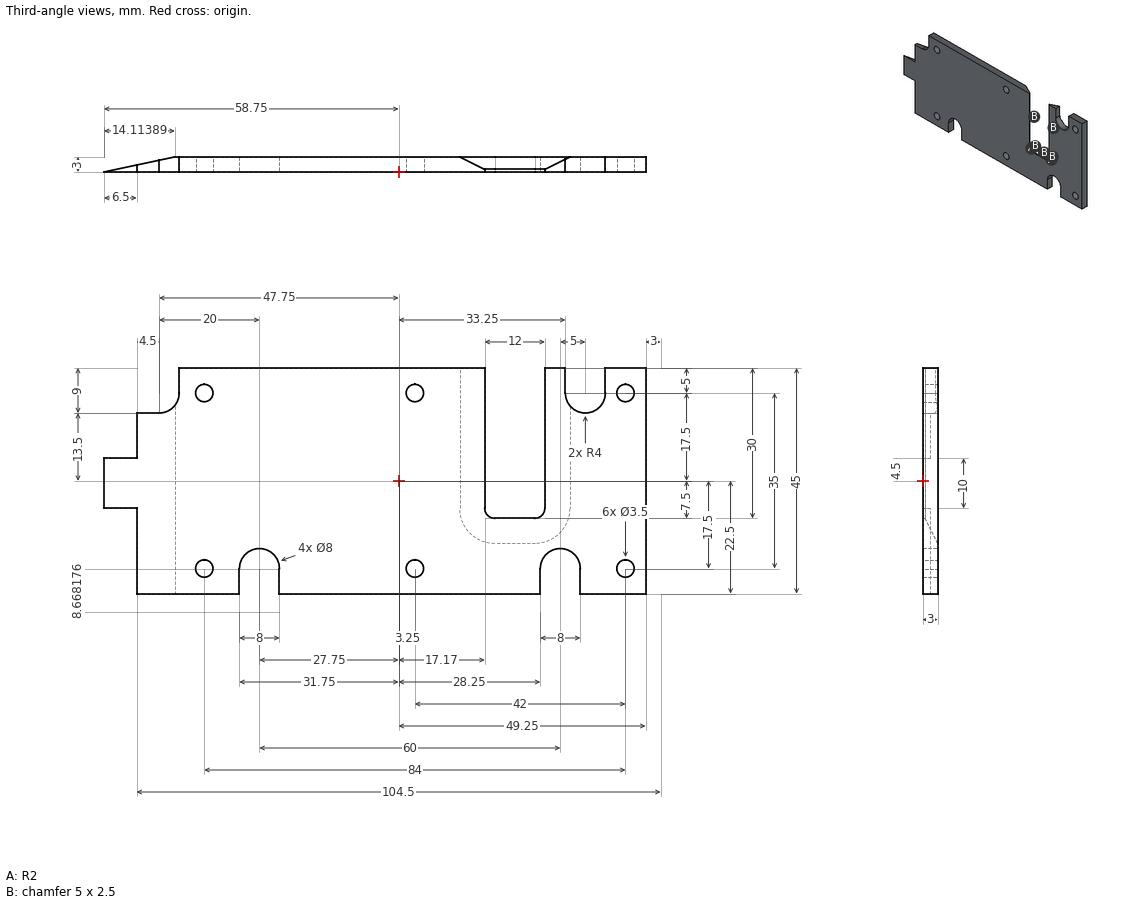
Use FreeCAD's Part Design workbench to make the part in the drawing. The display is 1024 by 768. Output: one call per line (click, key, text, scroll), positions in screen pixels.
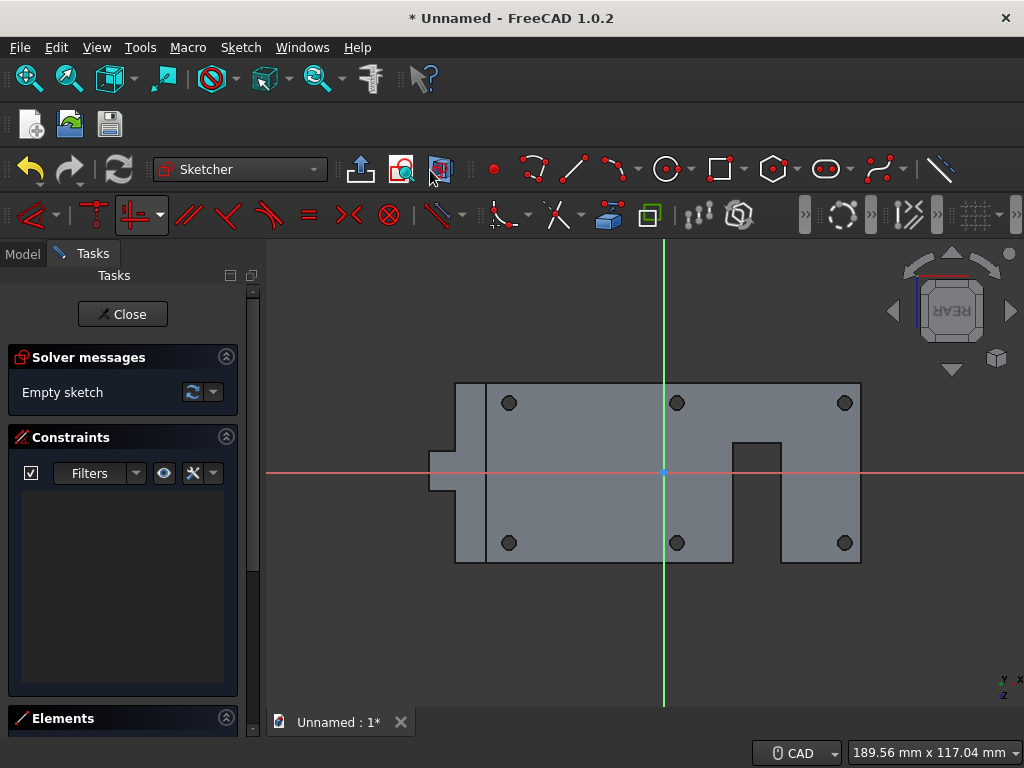
key(g)
key(c)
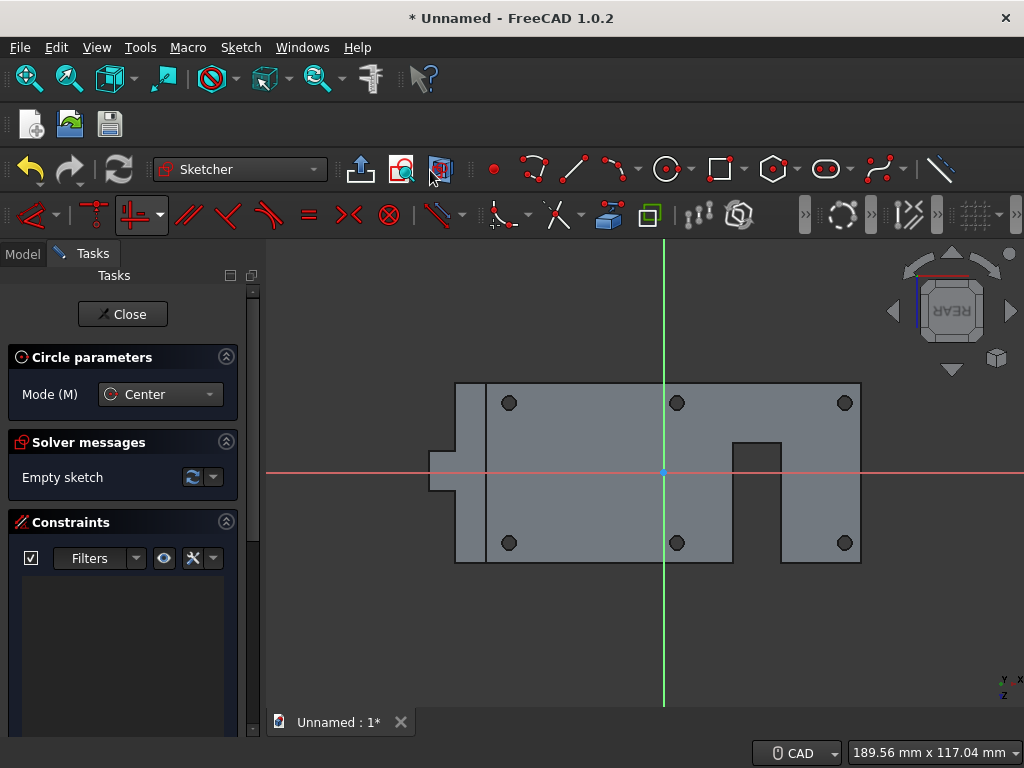
scroll(553, 403, up, 2)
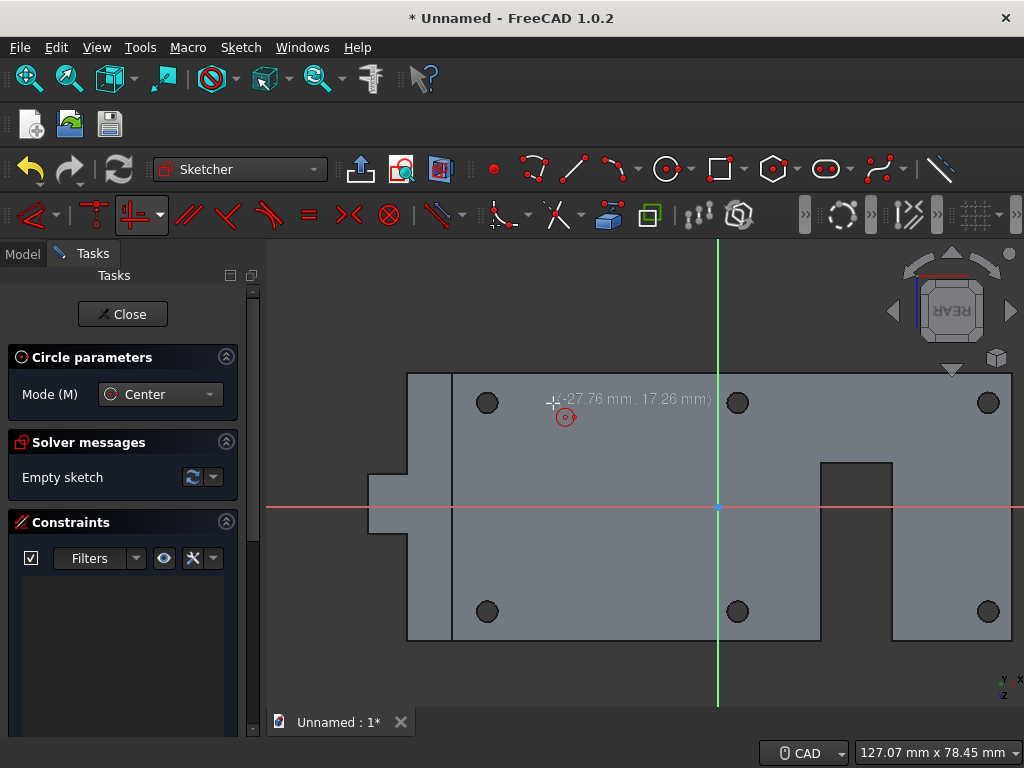
click(553, 403)
move(570, 386)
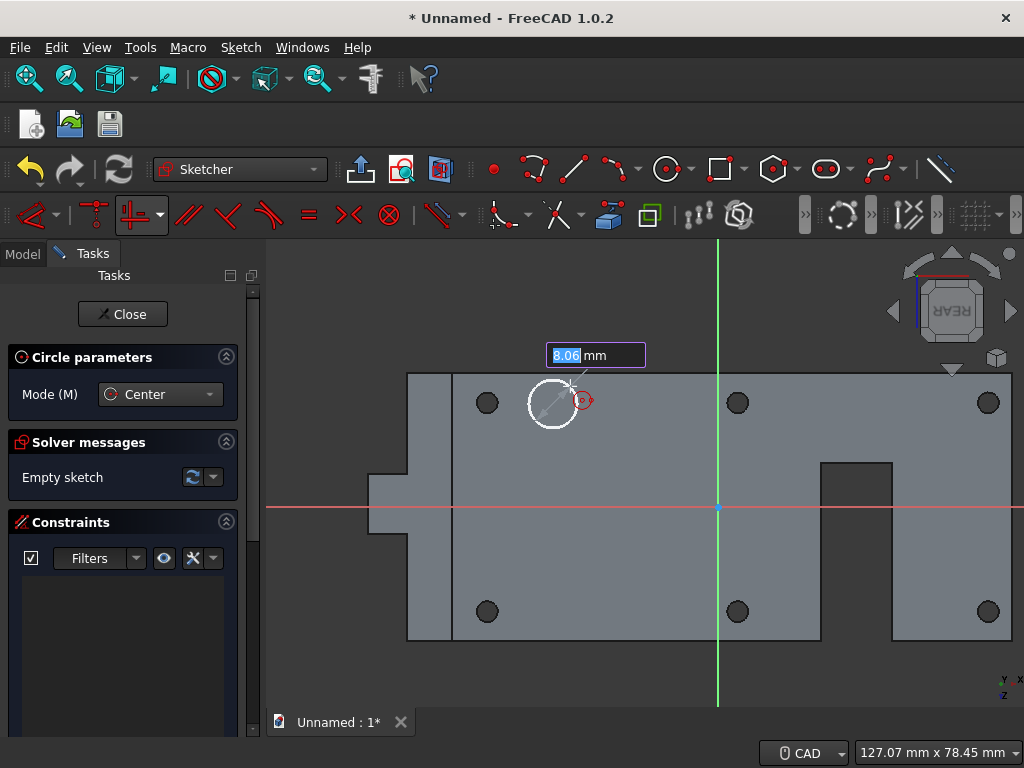
text(8)
key(Return)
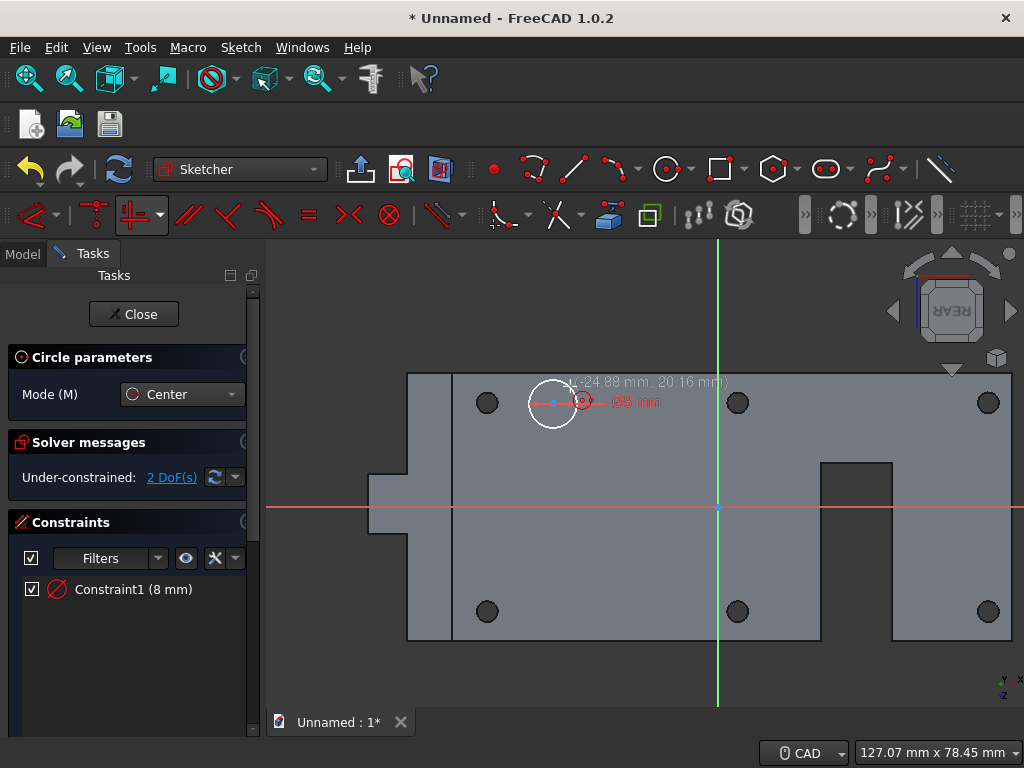
click(434, 612)
move(450, 595)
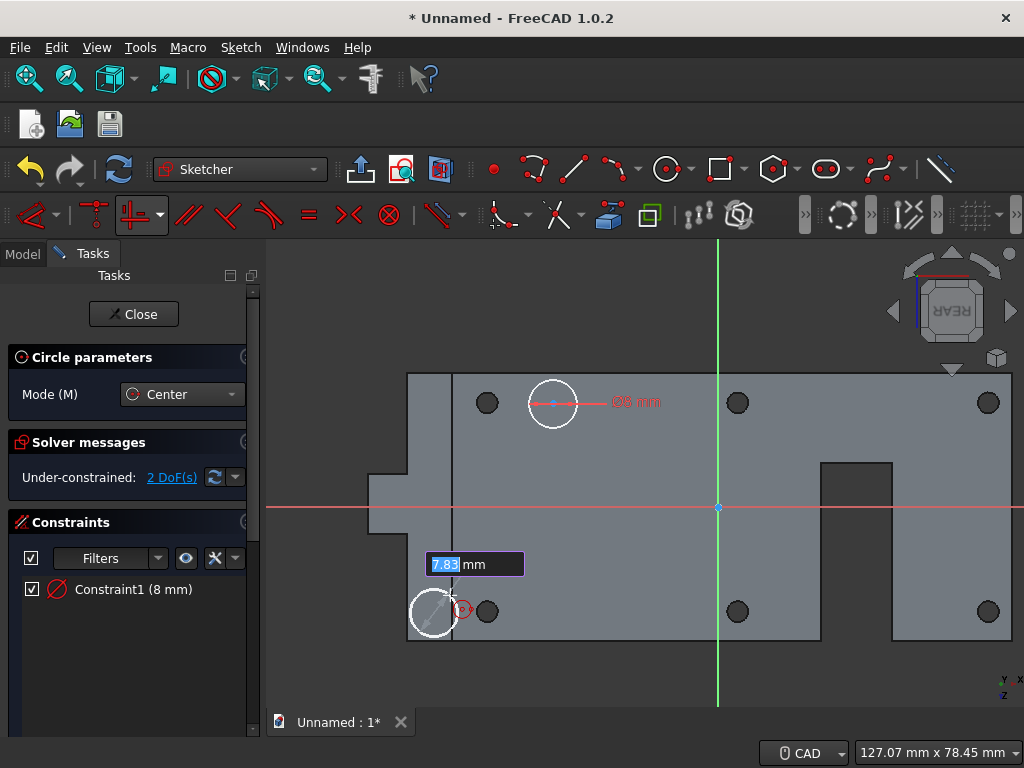
text(8)
key(Return)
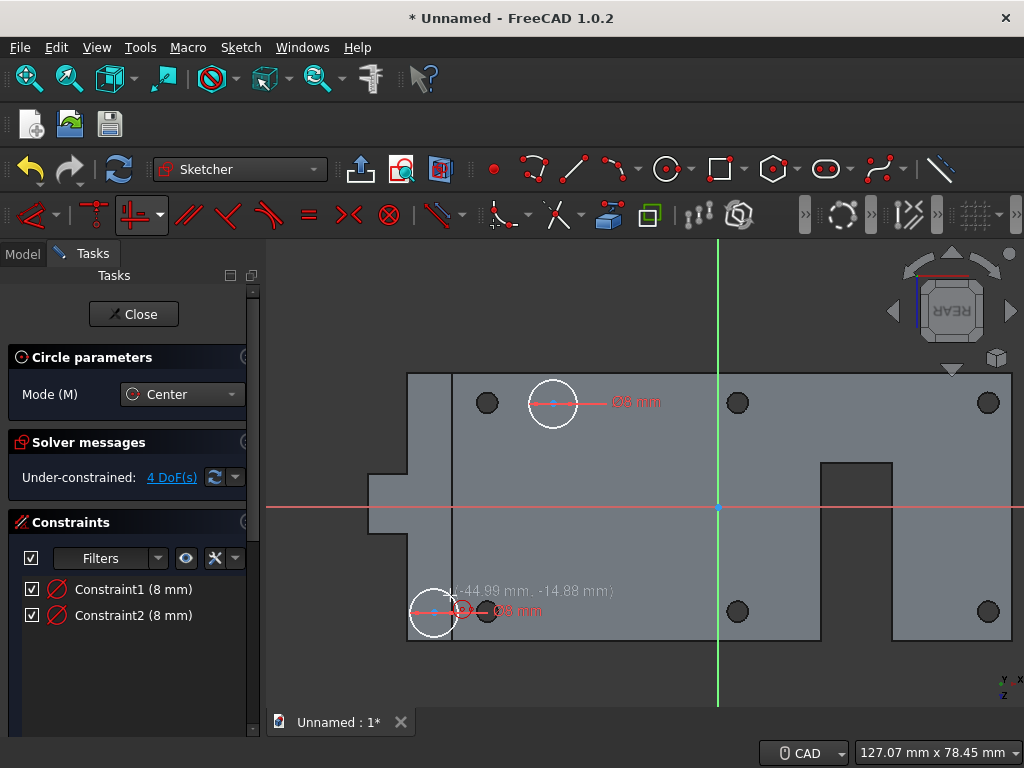
scroll(352, 403, down, 2)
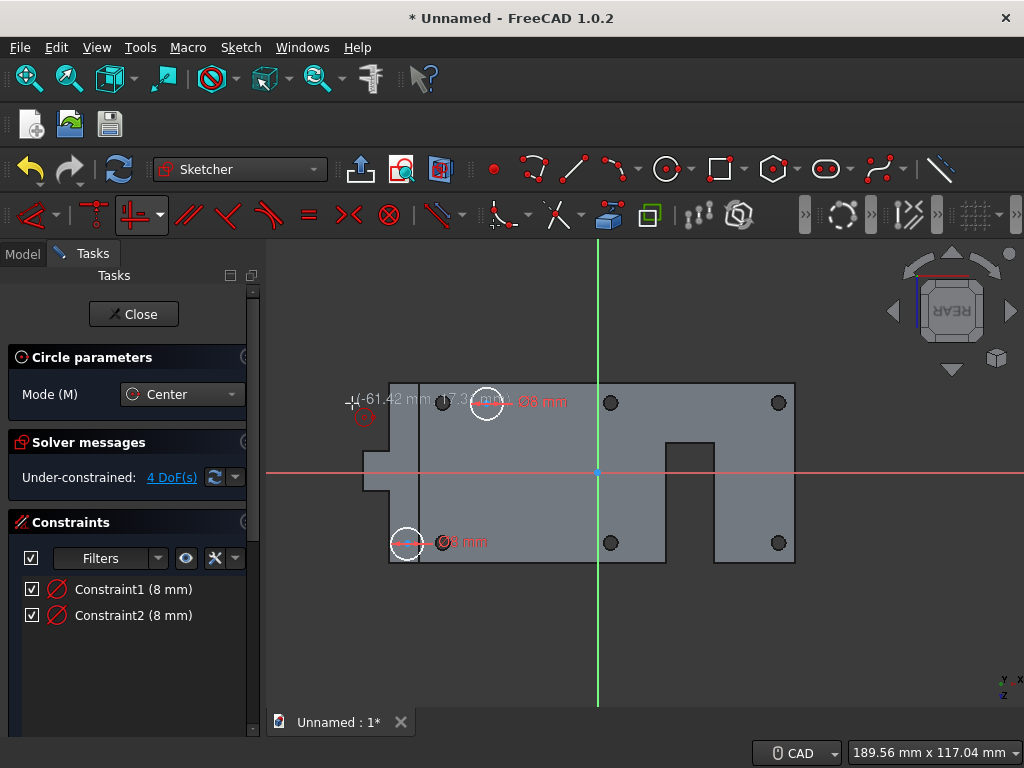
scroll(727, 403, up, 2)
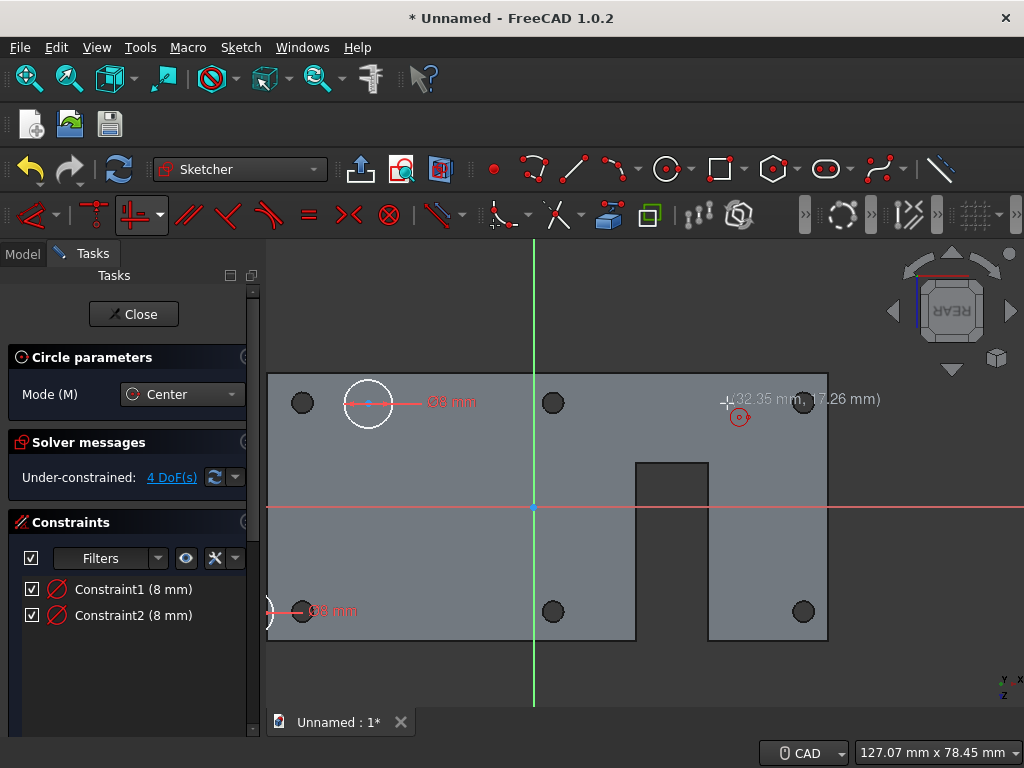
click(726, 403)
move(743, 386)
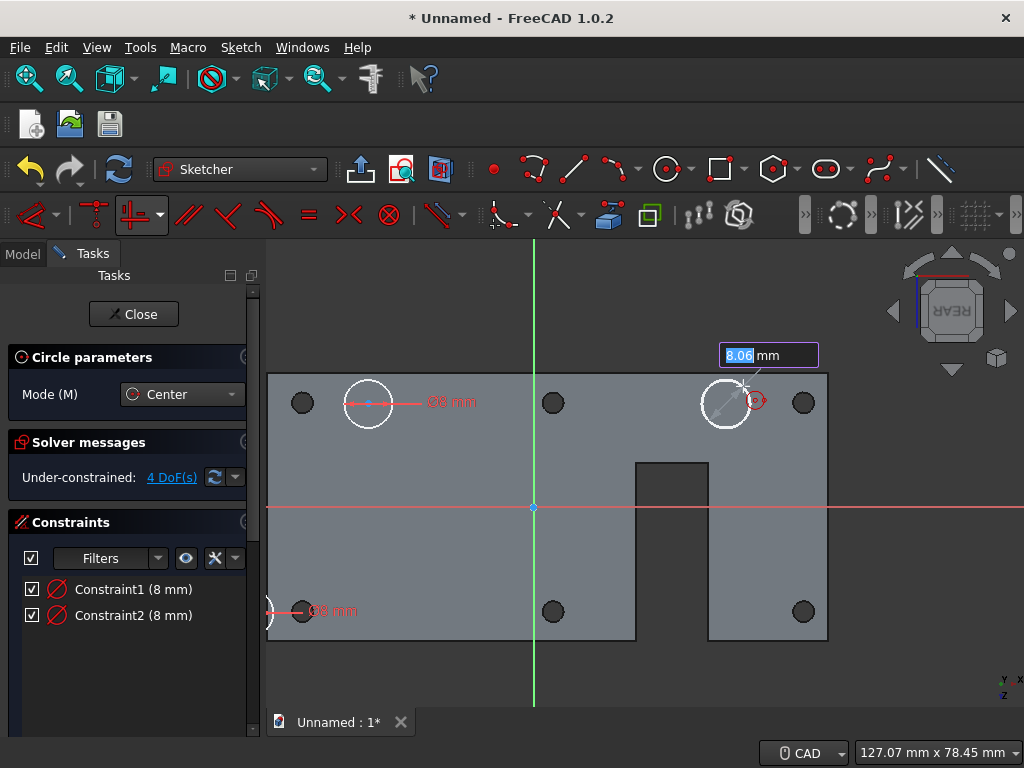
text(8)
key(Return)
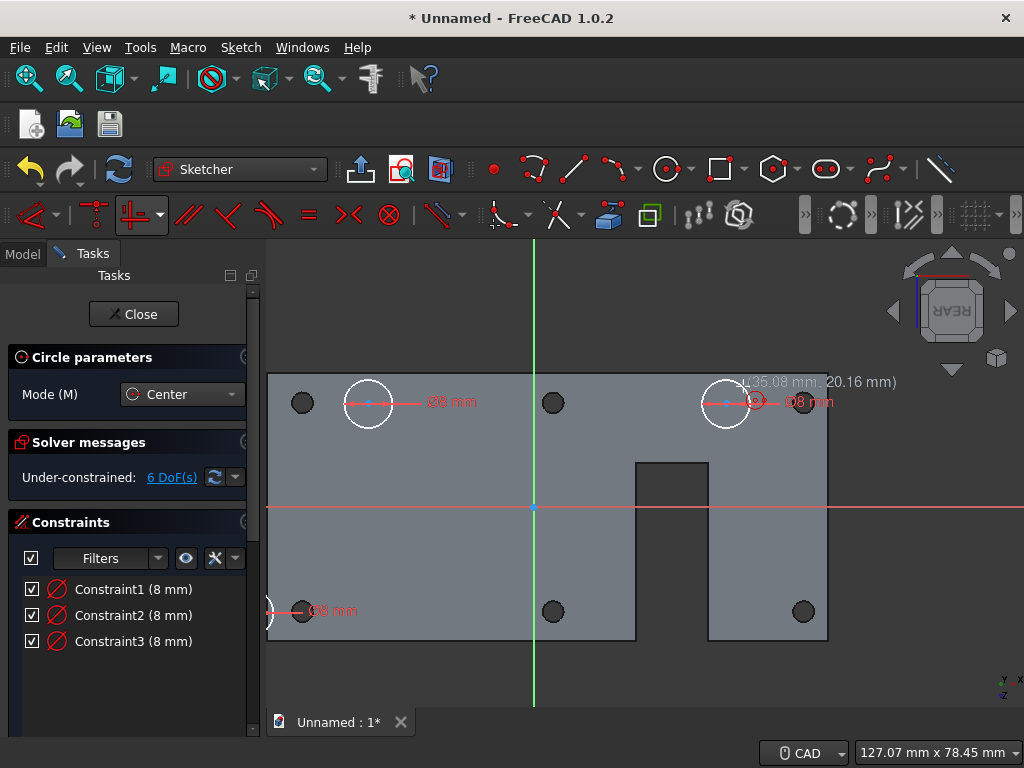
click(756, 612)
move(773, 595)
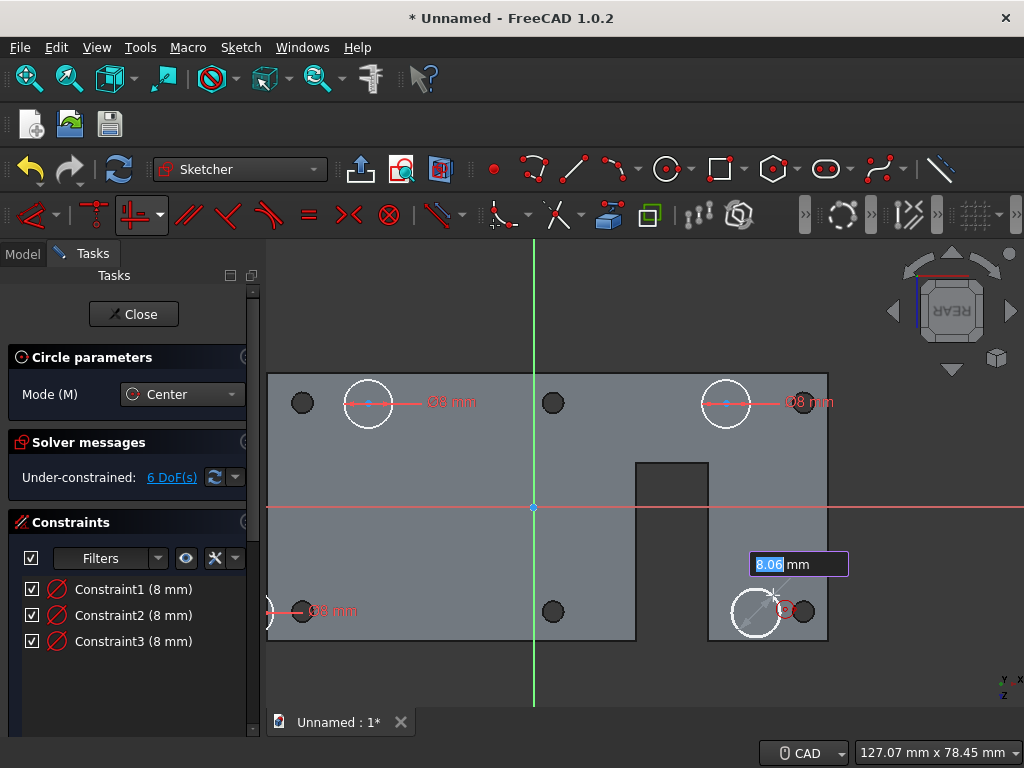
text(8)
key(Return)
key(Escape)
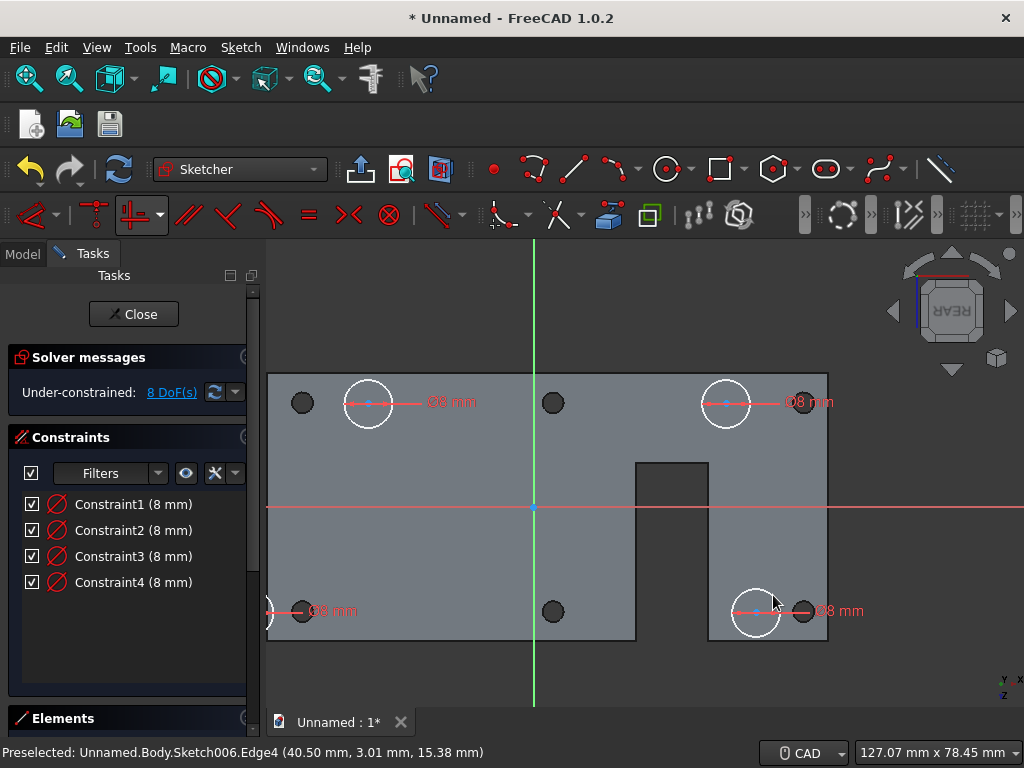
click(368, 404)